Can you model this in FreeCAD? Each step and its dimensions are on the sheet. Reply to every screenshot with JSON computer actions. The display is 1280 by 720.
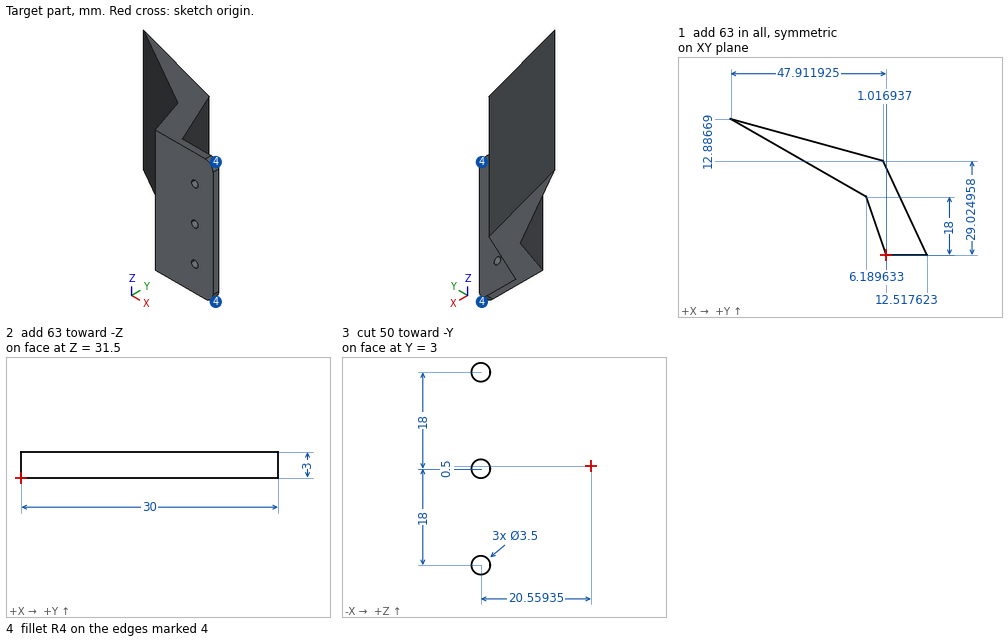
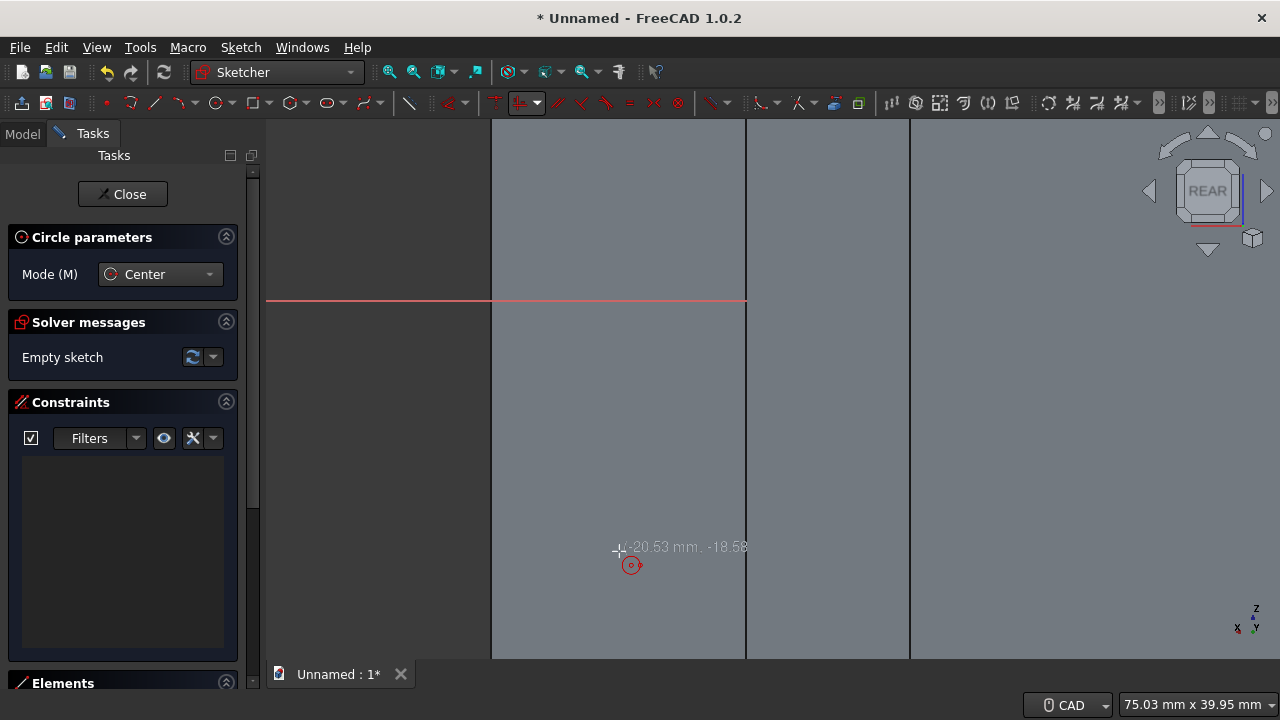
{"action": "left_click", "coordinate": [618, 551]}
{"action": "mouse_move", "coordinate": [635, 534]}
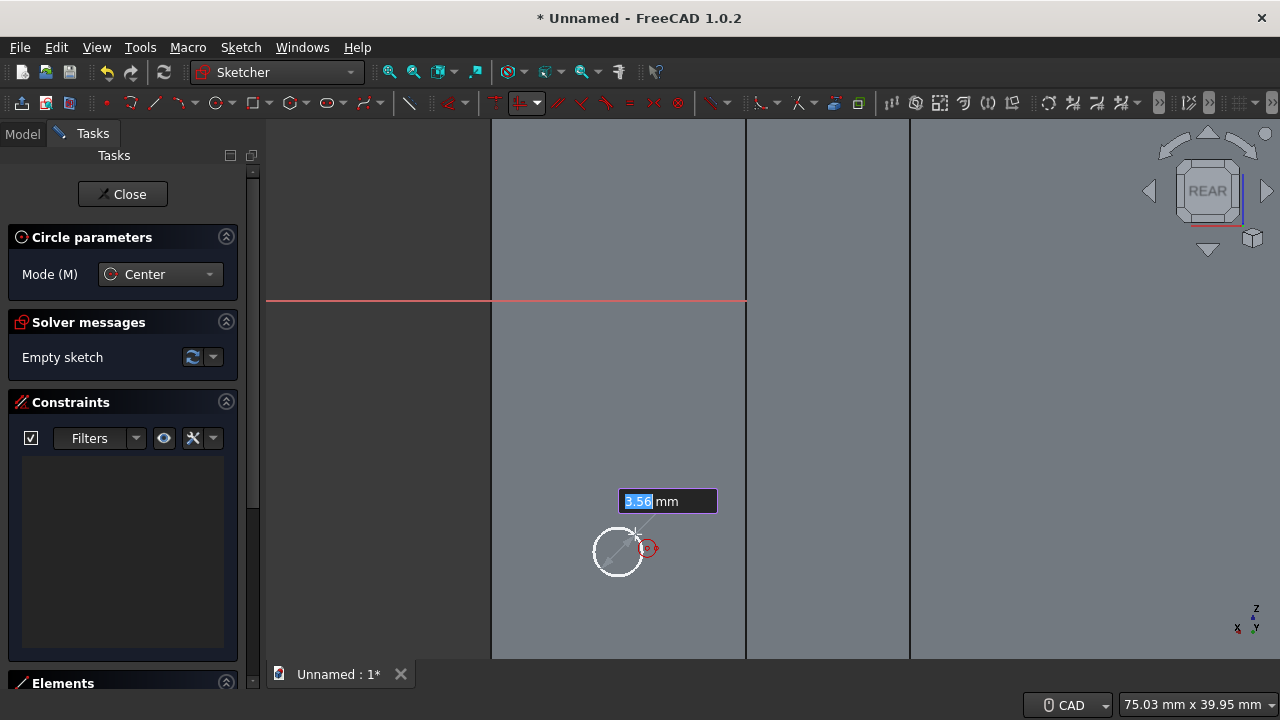
{"action": "type", "text": "3.5"}
{"action": "key", "text": "Return"}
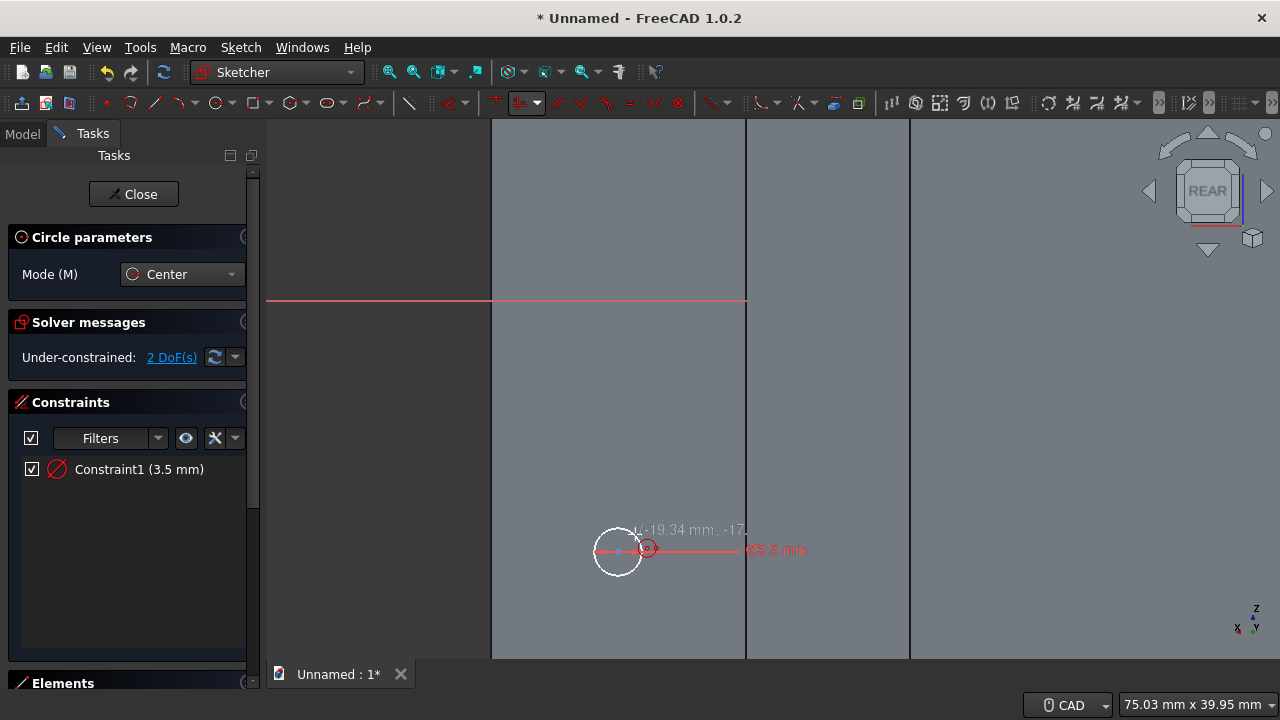
{"action": "scroll", "coordinate": [618, 308], "scroll_direction": "up", "scroll_amount": 5}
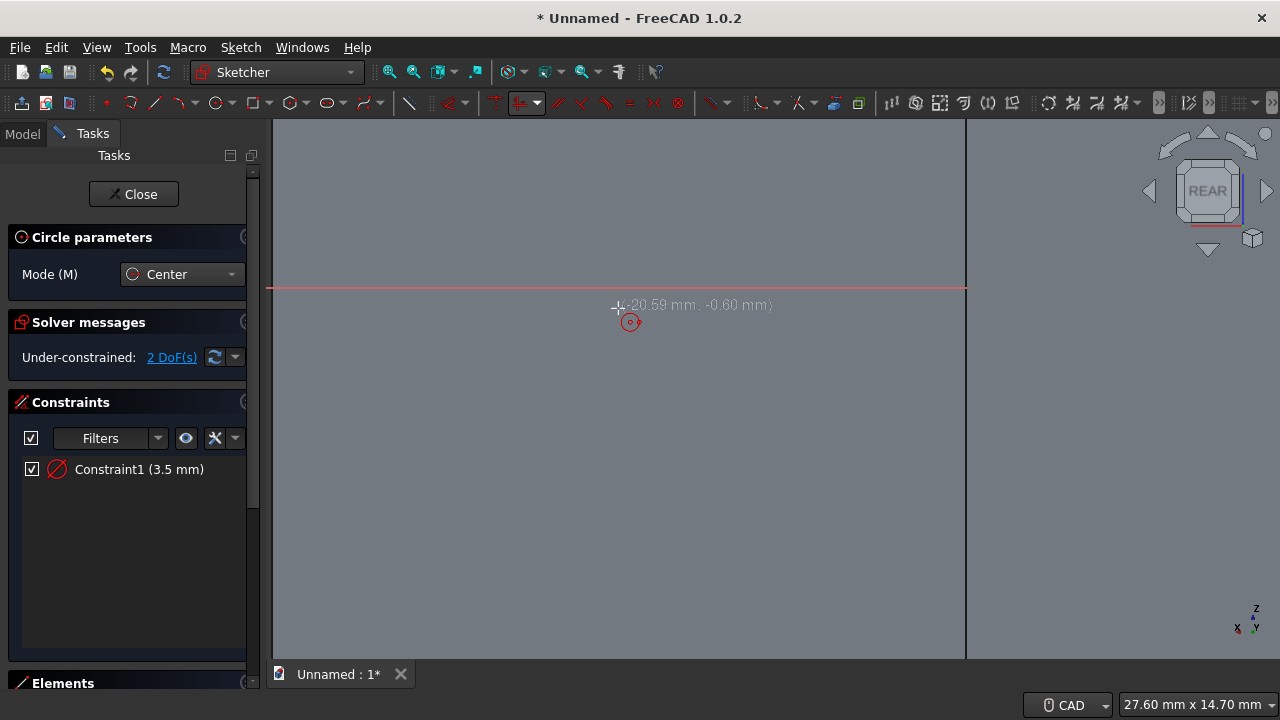
{"action": "left_click", "coordinate": [619, 307]}
{"action": "mouse_move", "coordinate": [664, 261]}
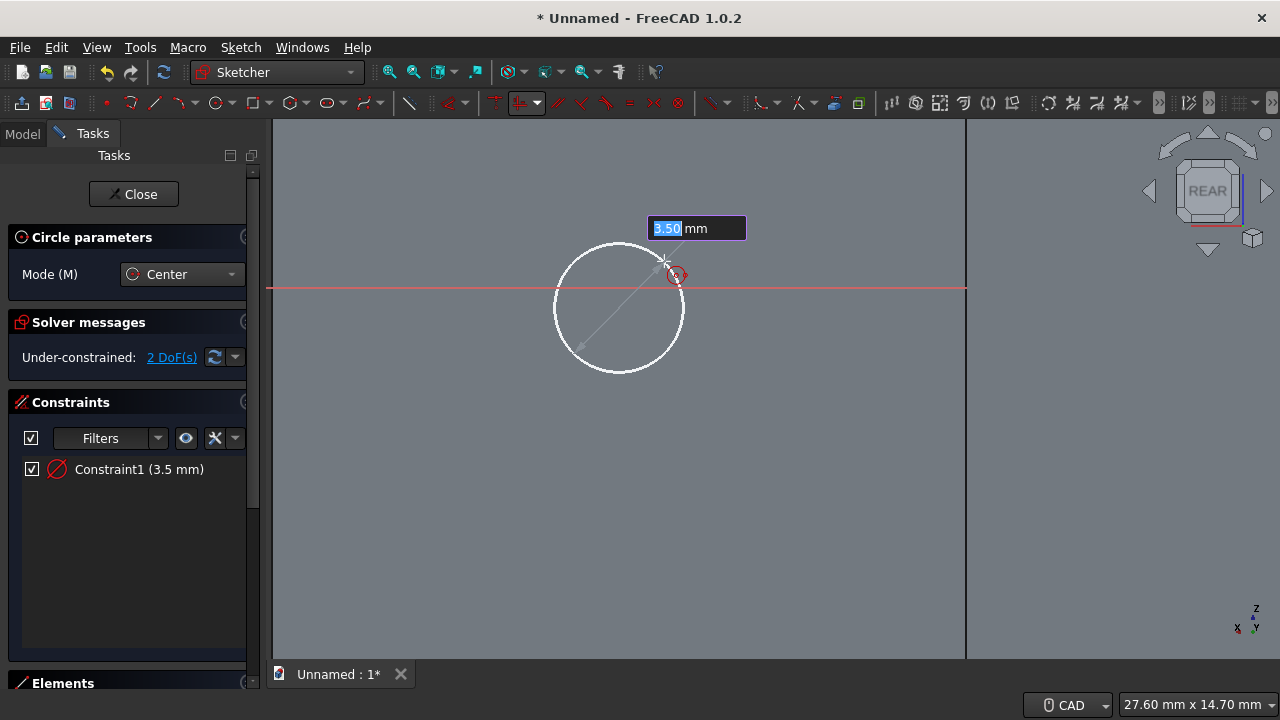
{"action": "type", "text": "3.5"}
{"action": "key", "text": "Return"}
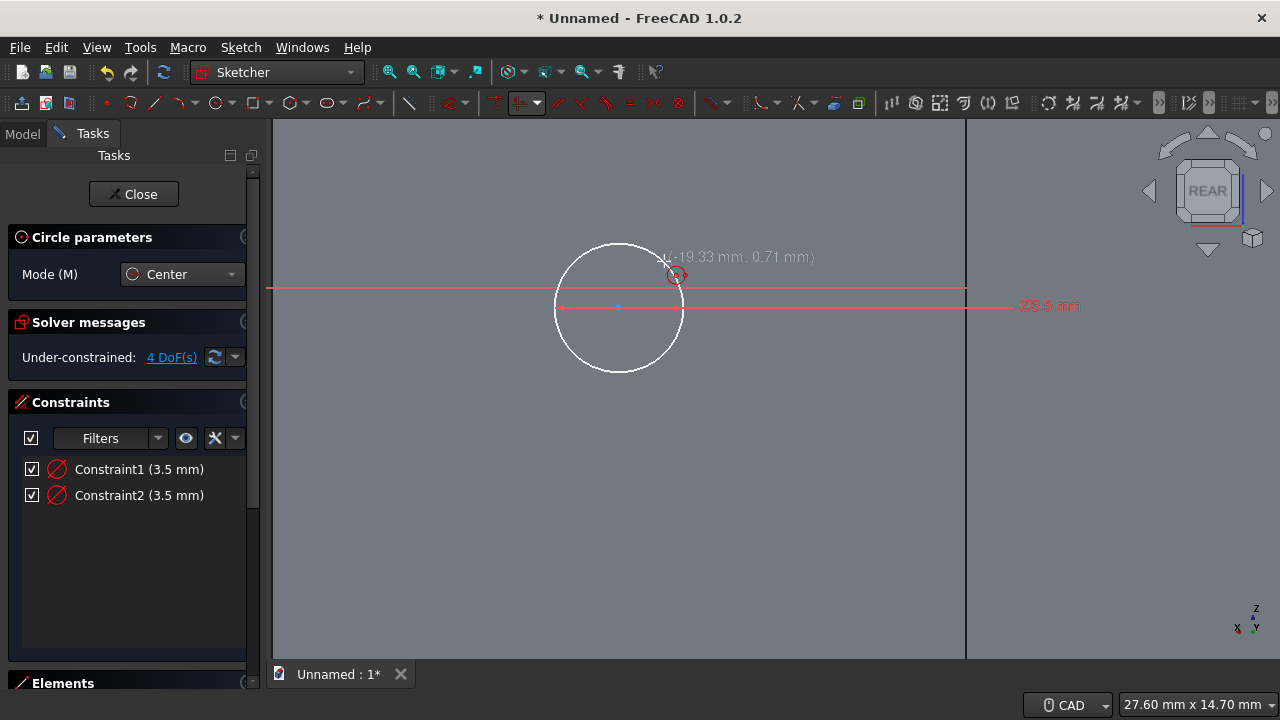
{"action": "scroll", "coordinate": [620, 416], "scroll_direction": "down", "scroll_amount": 7}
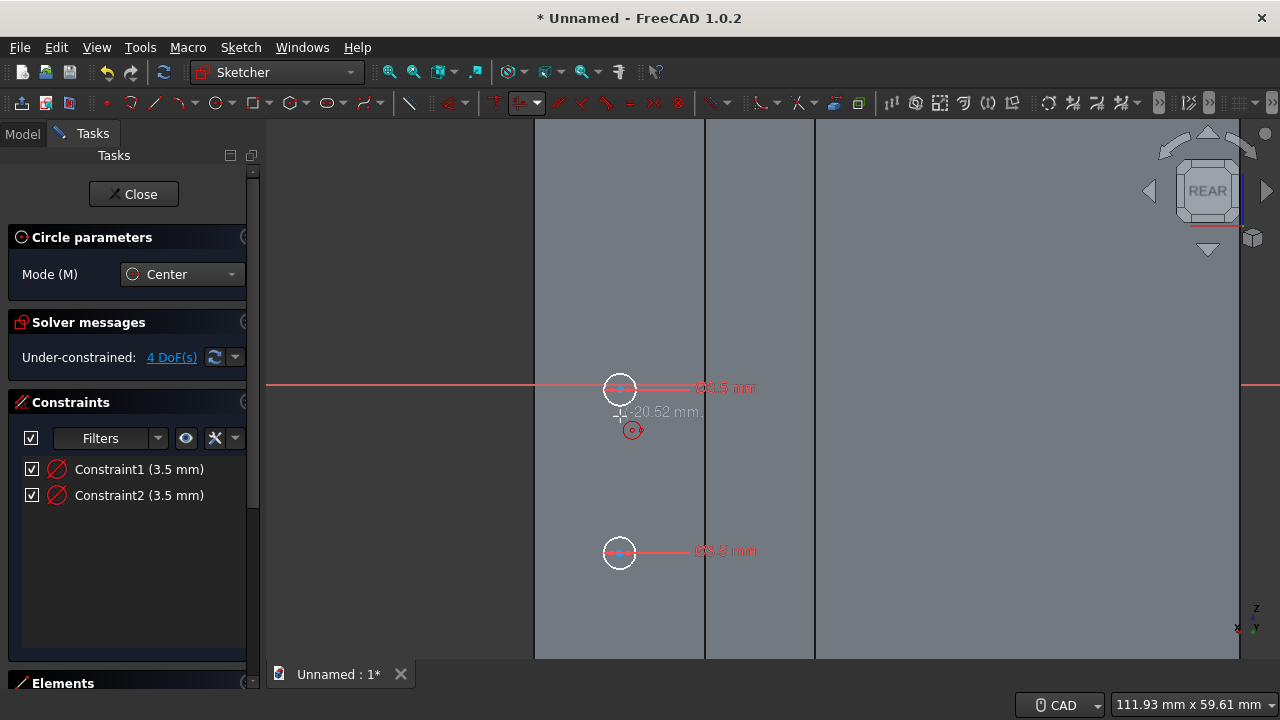
{"action": "scroll", "coordinate": [620, 226], "scroll_direction": "up", "scroll_amount": 2}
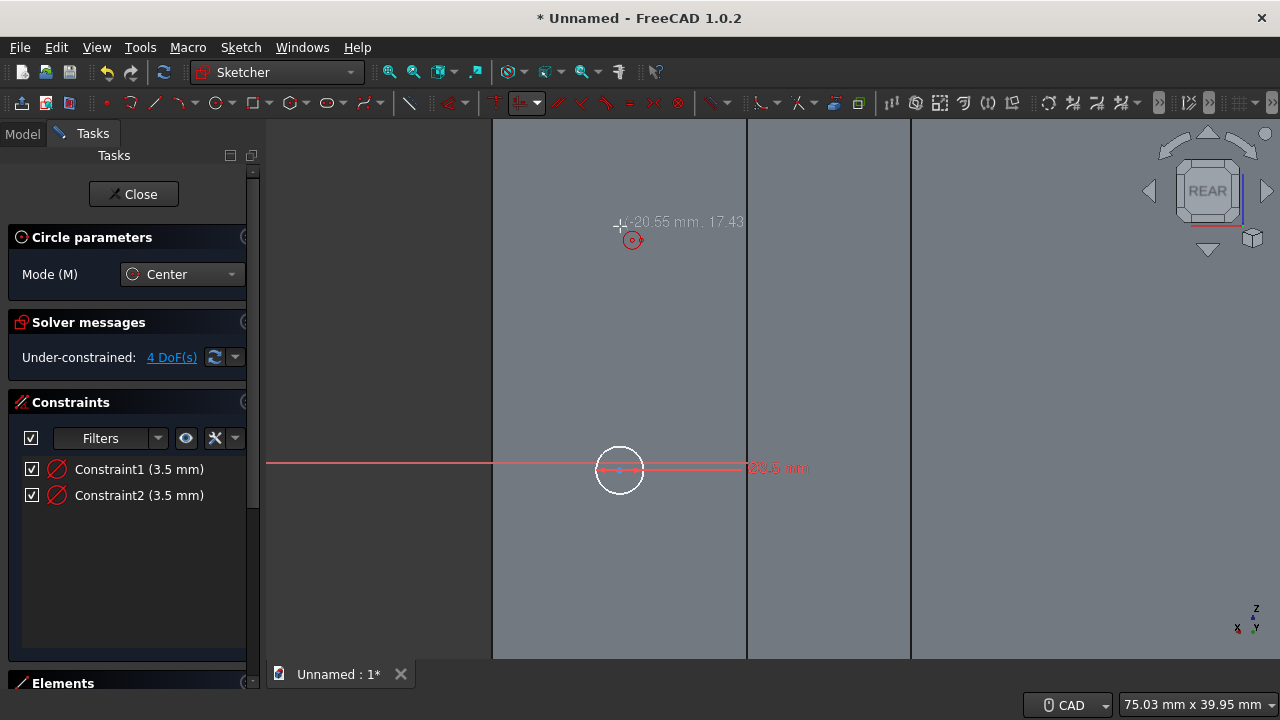
{"action": "left_click", "coordinate": [620, 226]}
{"action": "mouse_move", "coordinate": [636, 210]}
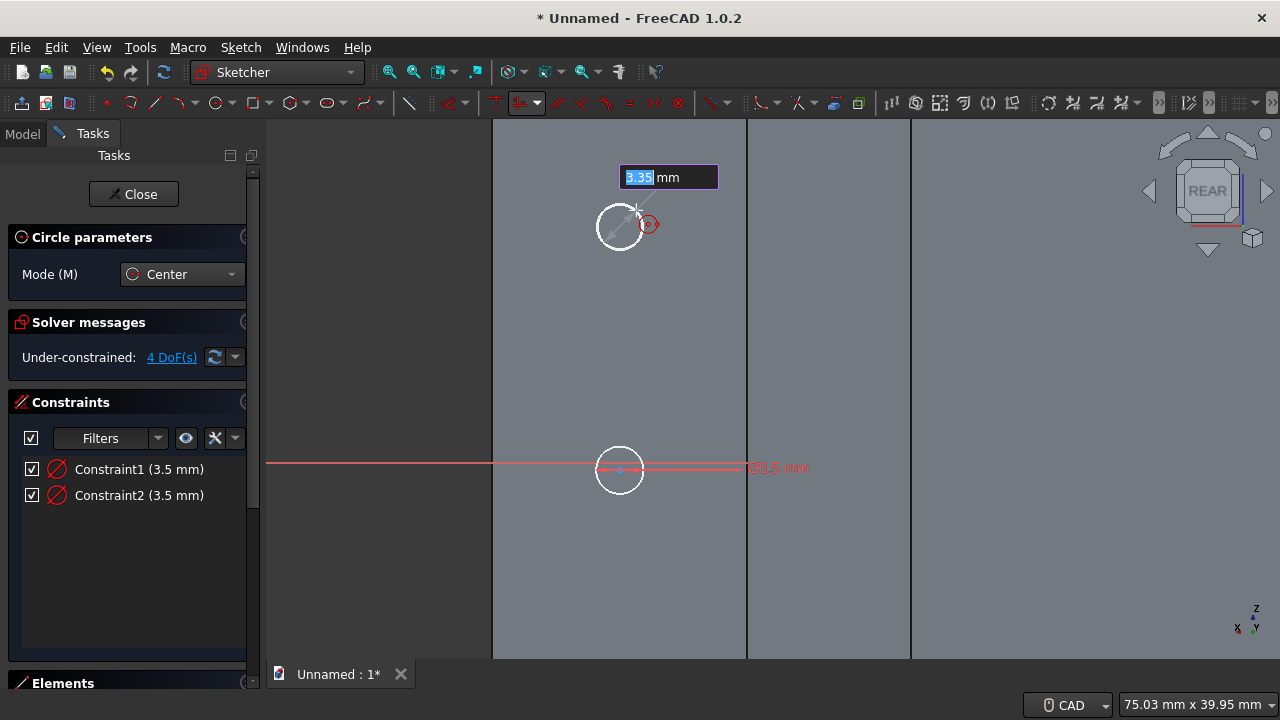
{"action": "type", "text": "3.5"}
{"action": "key", "text": "Return"}
{"action": "key", "text": "Escape"}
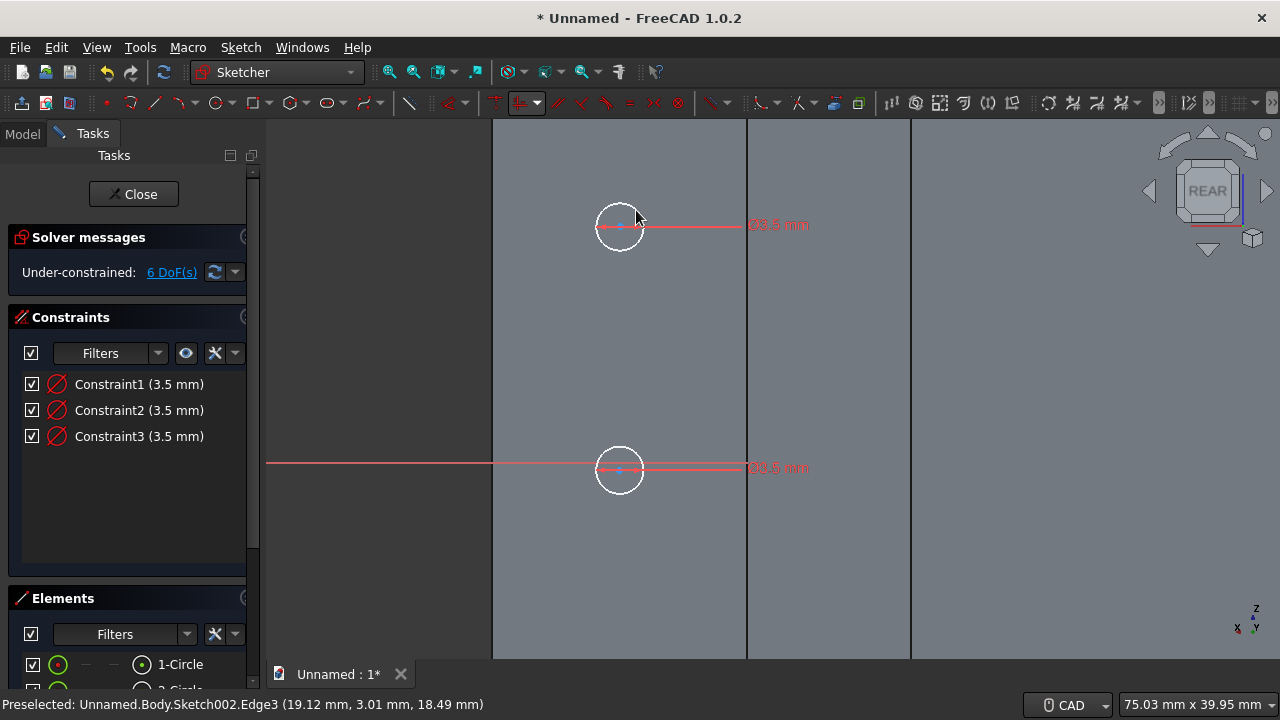
{"action": "scroll", "coordinate": [618, 225], "scroll_direction": "down", "scroll_amount": 2}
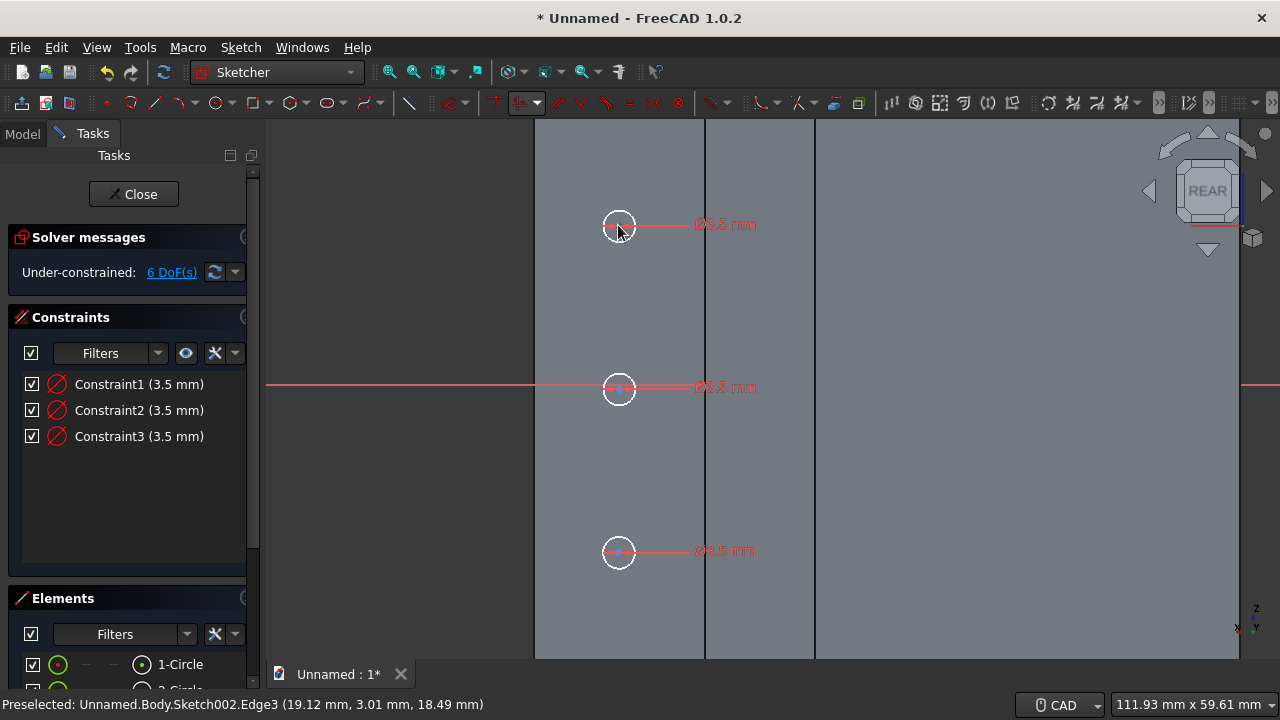
{"action": "left_click", "coordinate": [619, 553]}